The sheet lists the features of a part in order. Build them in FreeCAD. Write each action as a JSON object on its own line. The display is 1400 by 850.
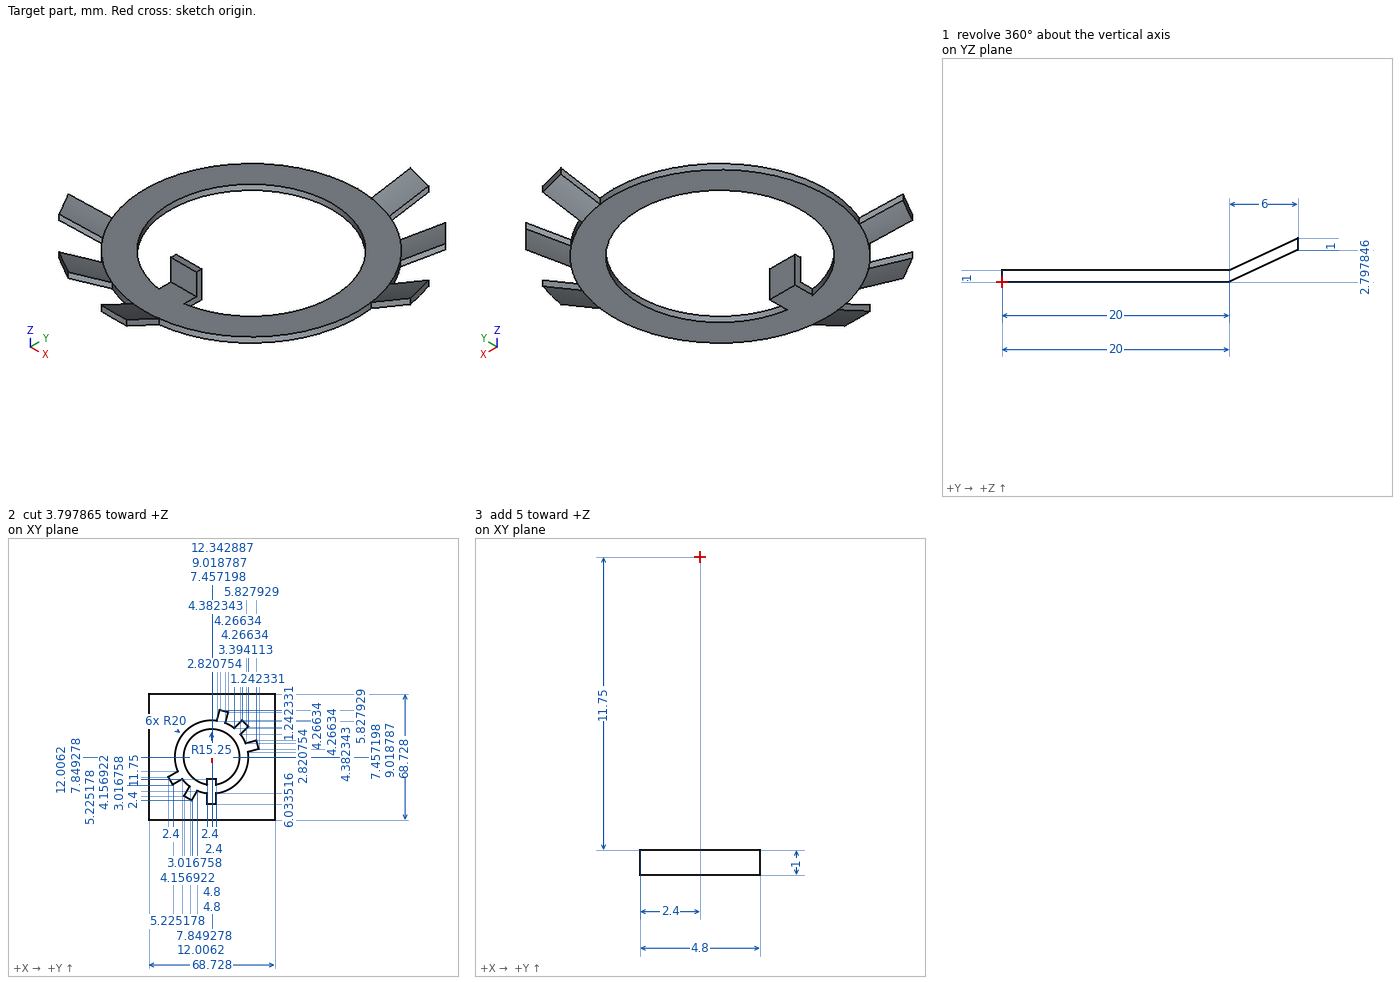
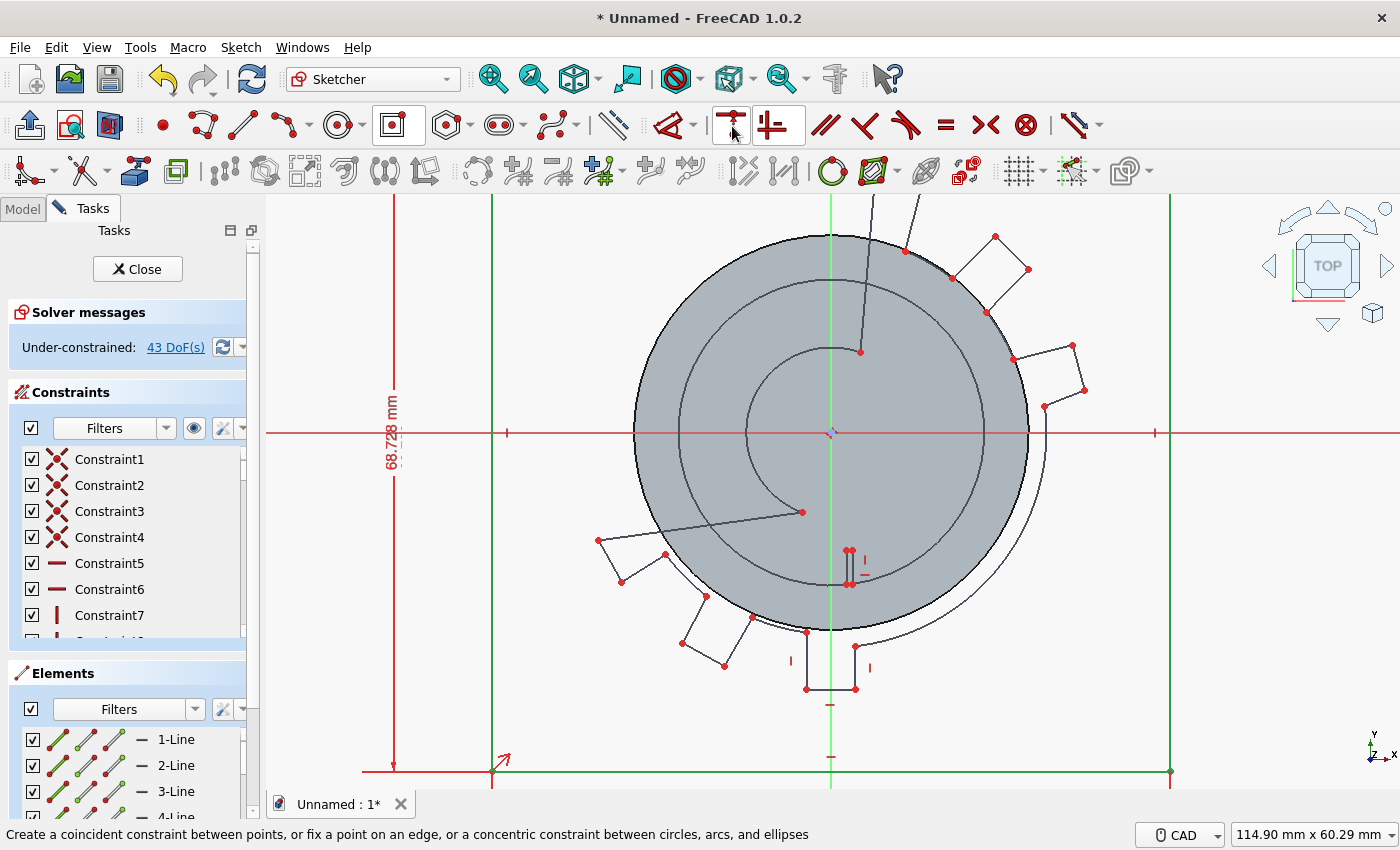
{"action": "left_click", "coordinate": [677, 568]}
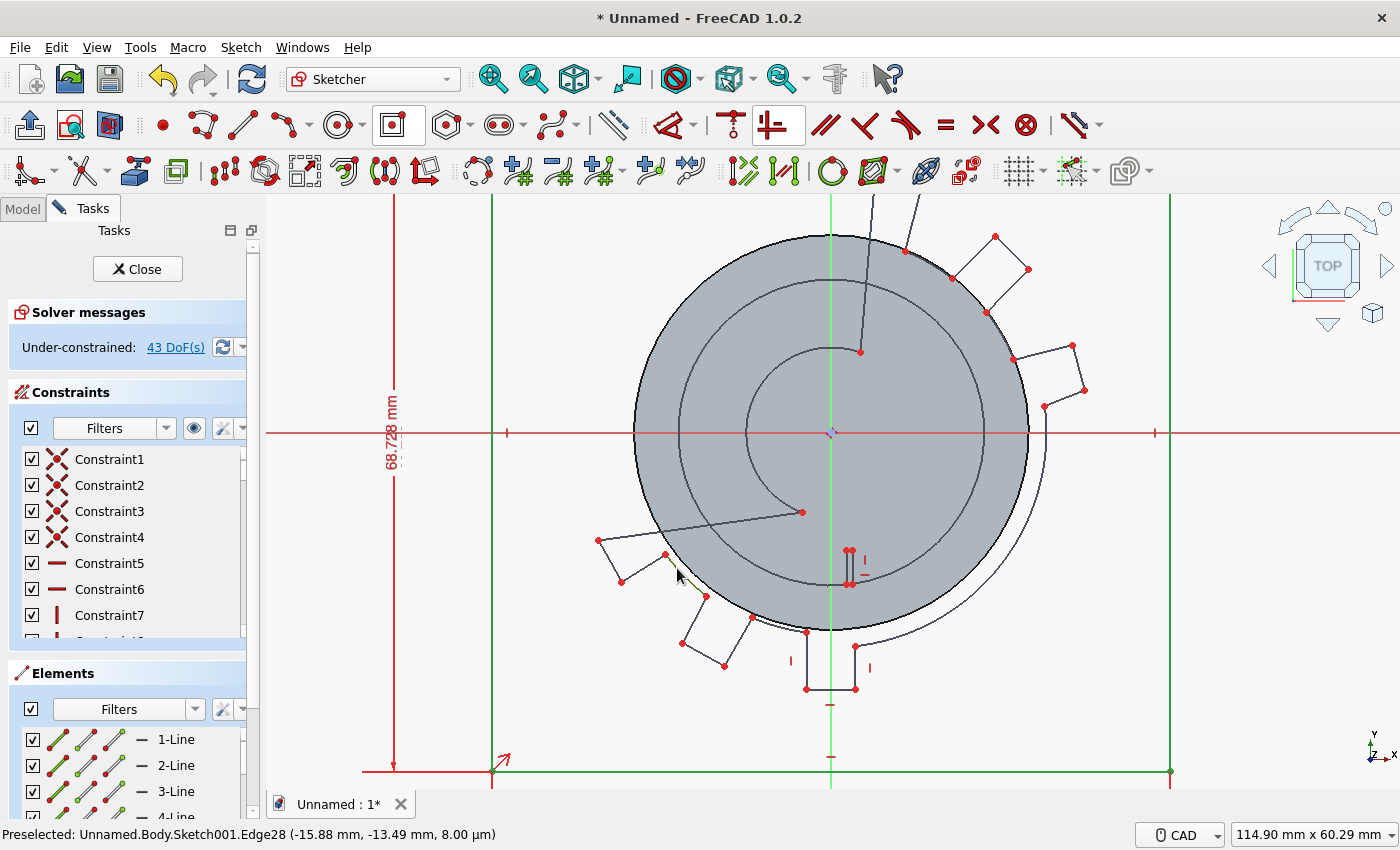
{"action": "left_click", "coordinate": [784, 362]}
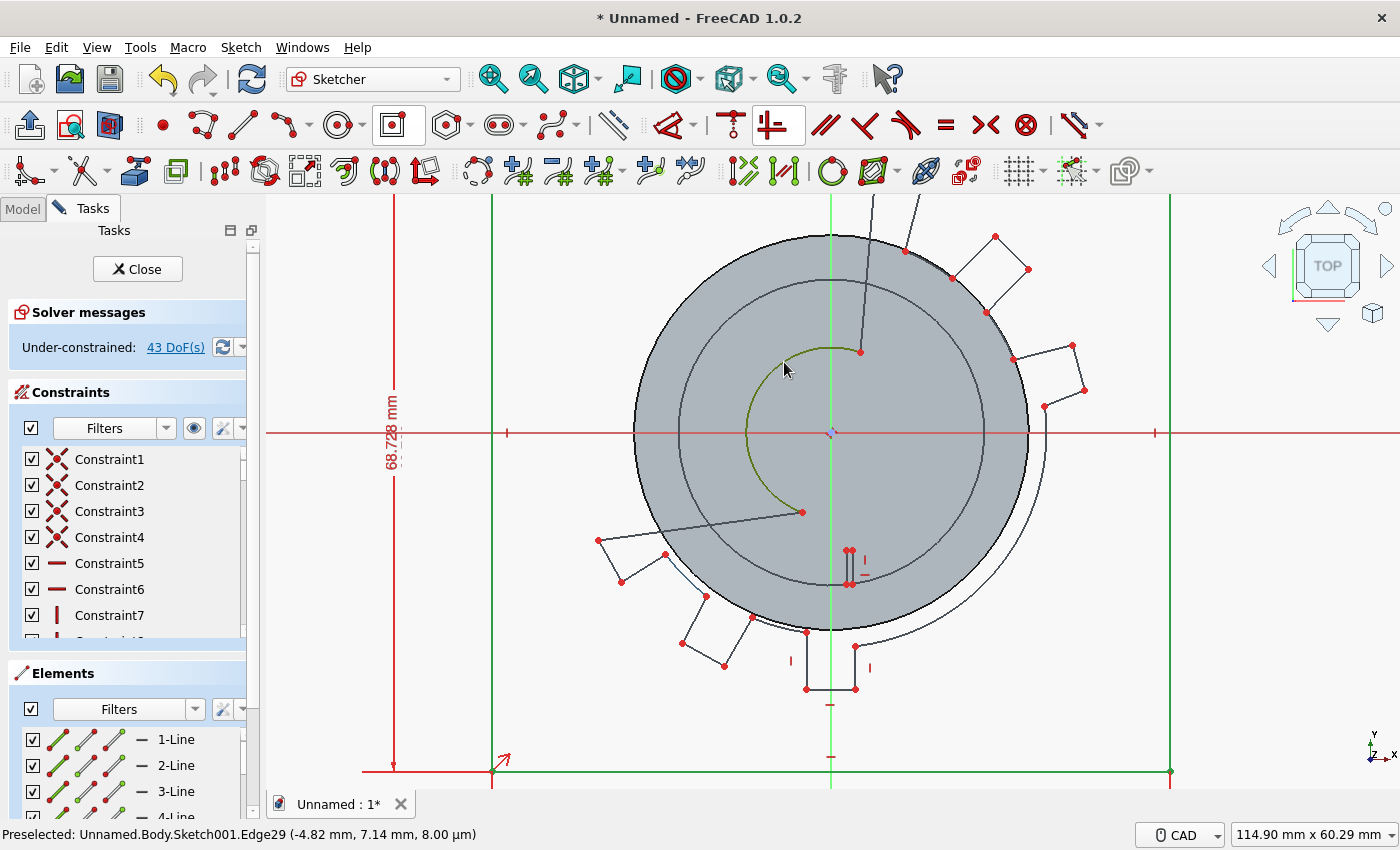
{"action": "left_click", "coordinate": [939, 269]}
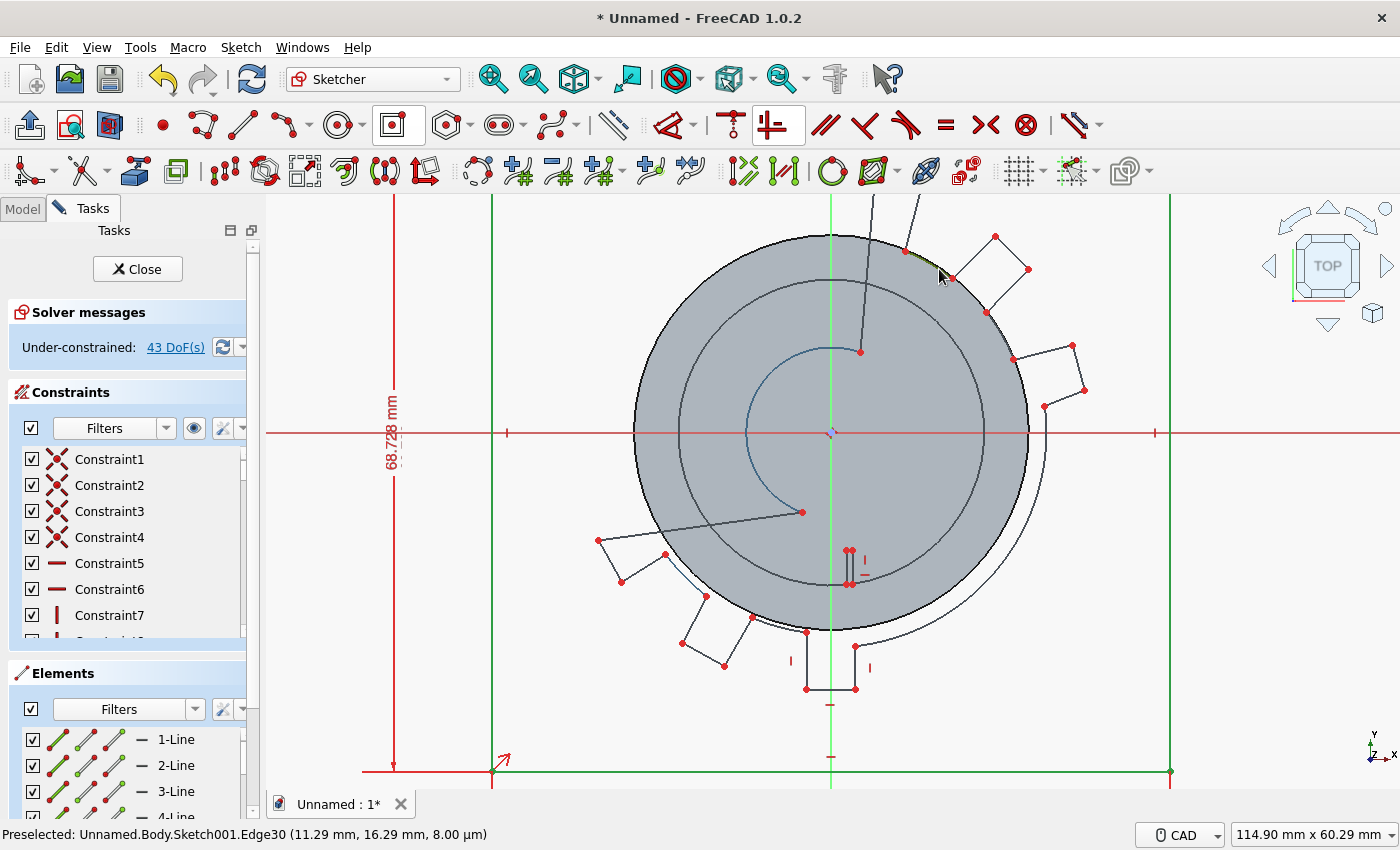
{"action": "left_click", "coordinate": [1007, 345]}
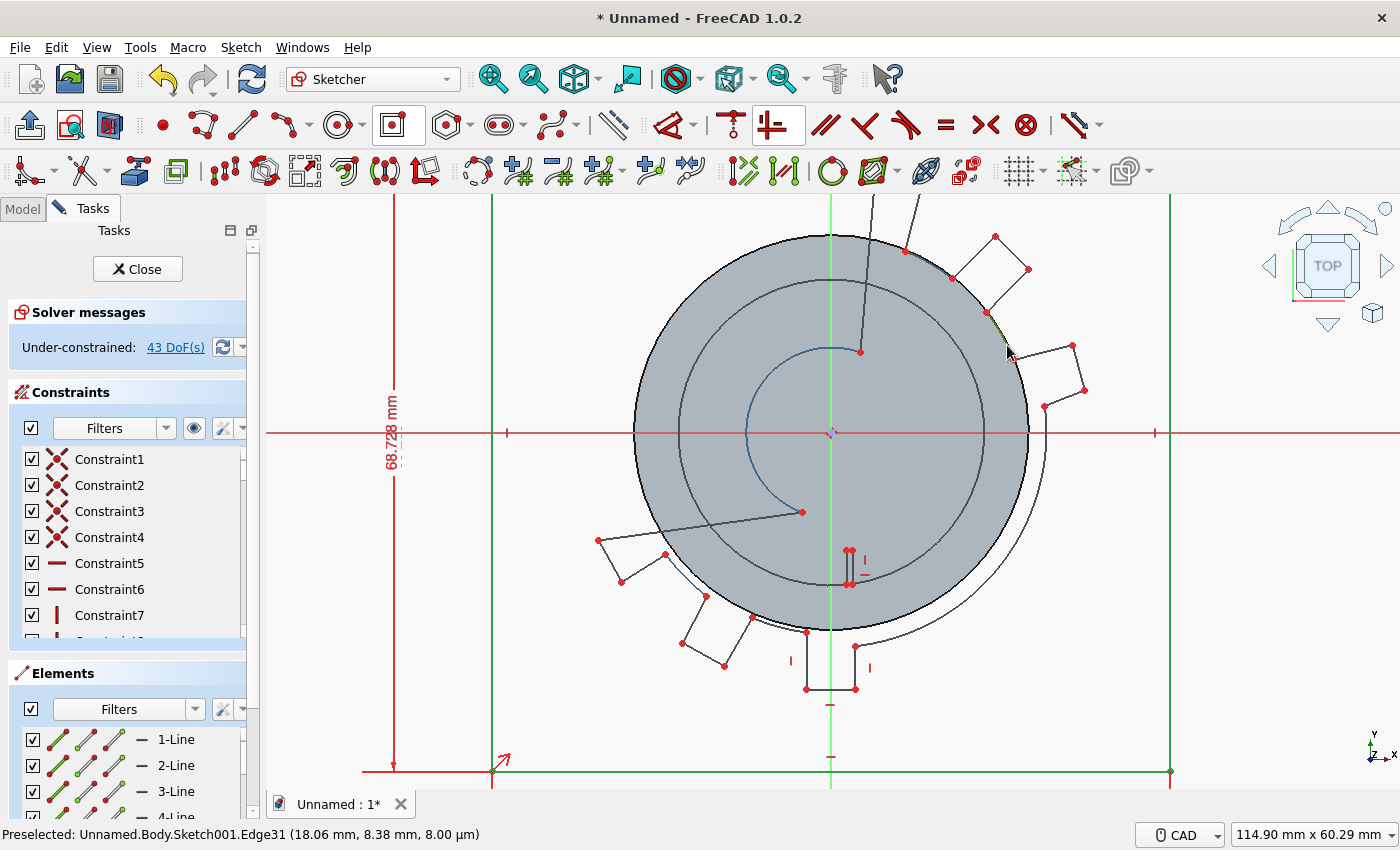
{"action": "left_click", "coordinate": [950, 612]}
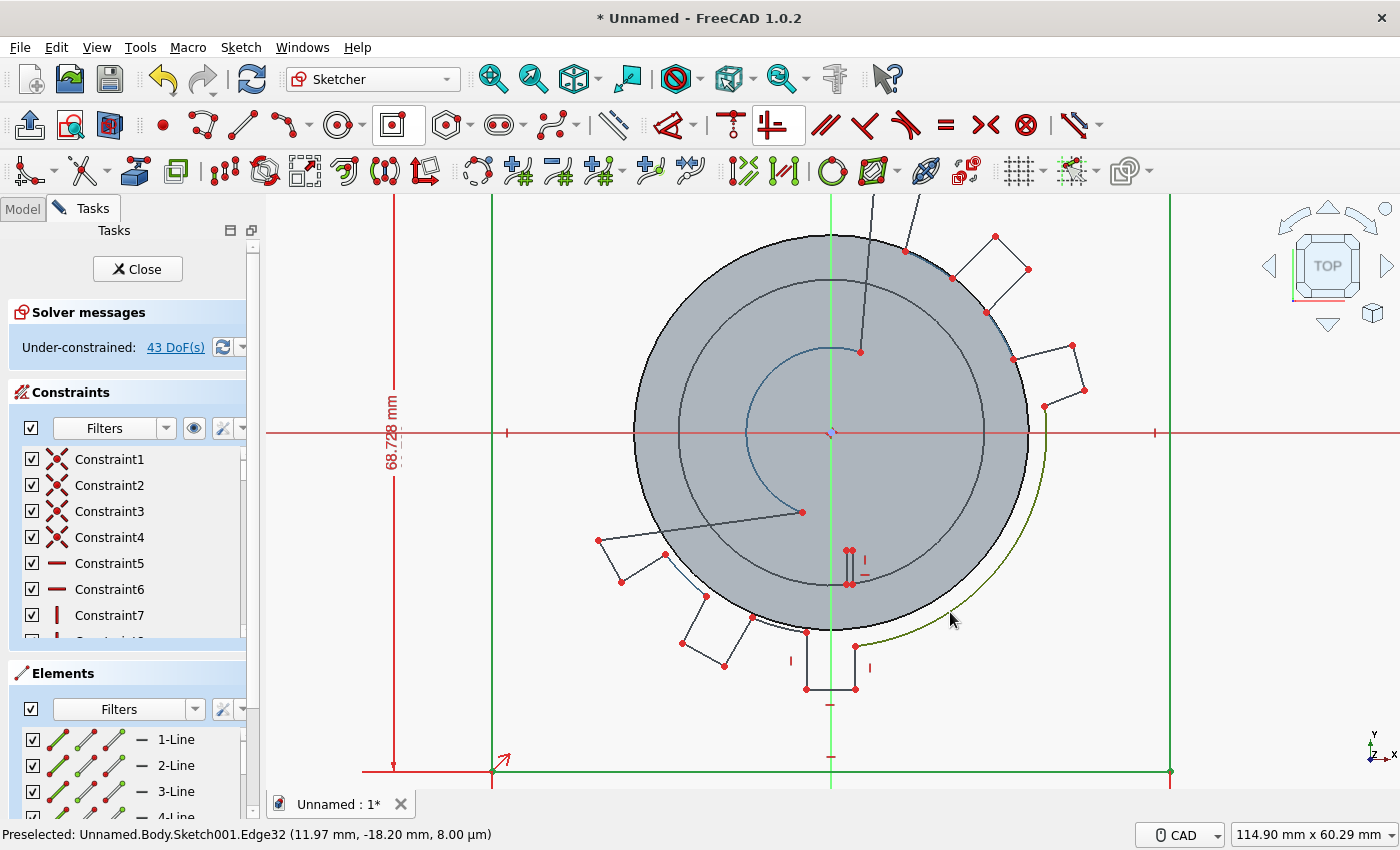
{"action": "left_click", "coordinate": [768, 624]}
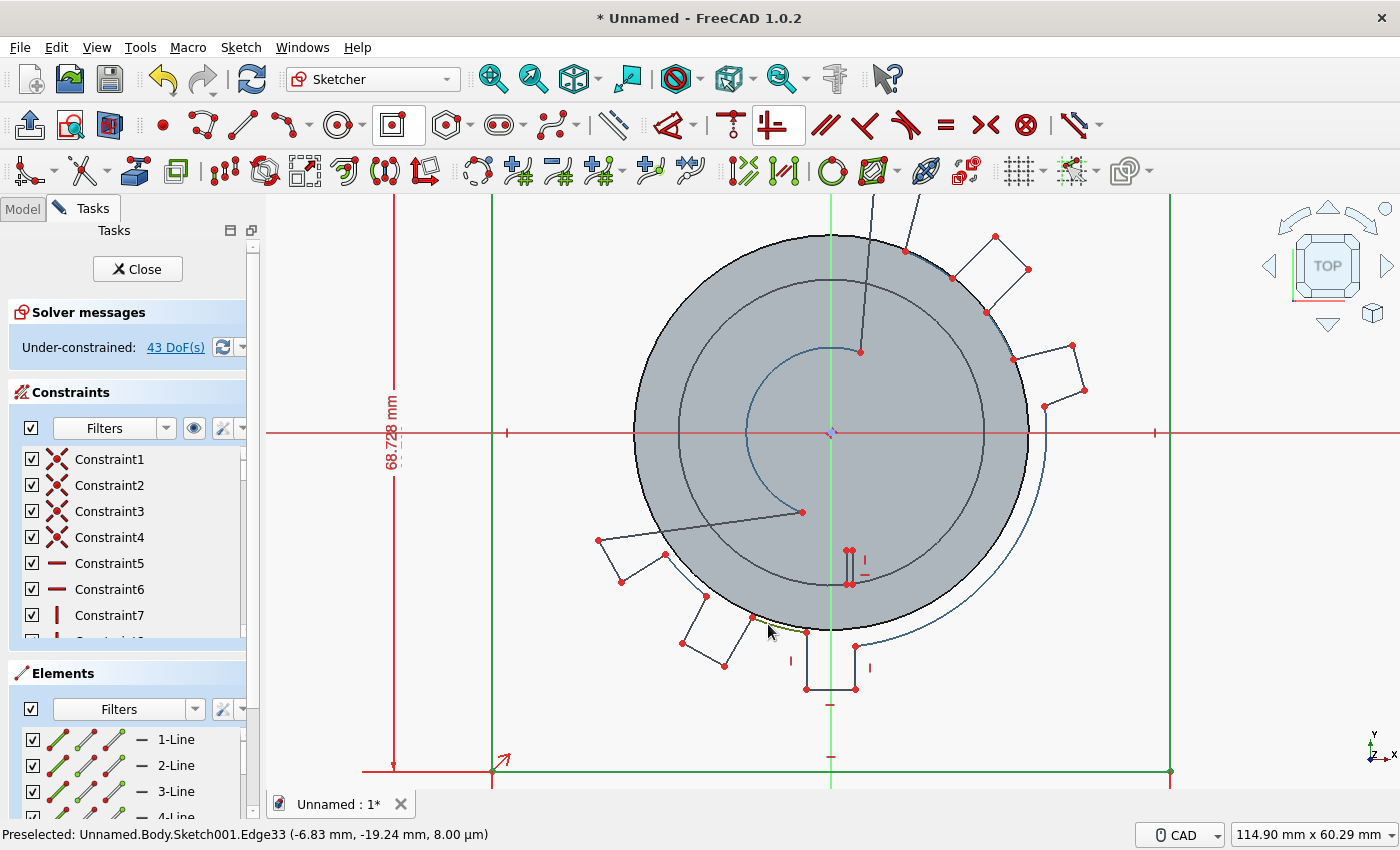
{"action": "left_click", "coordinate": [946, 126]}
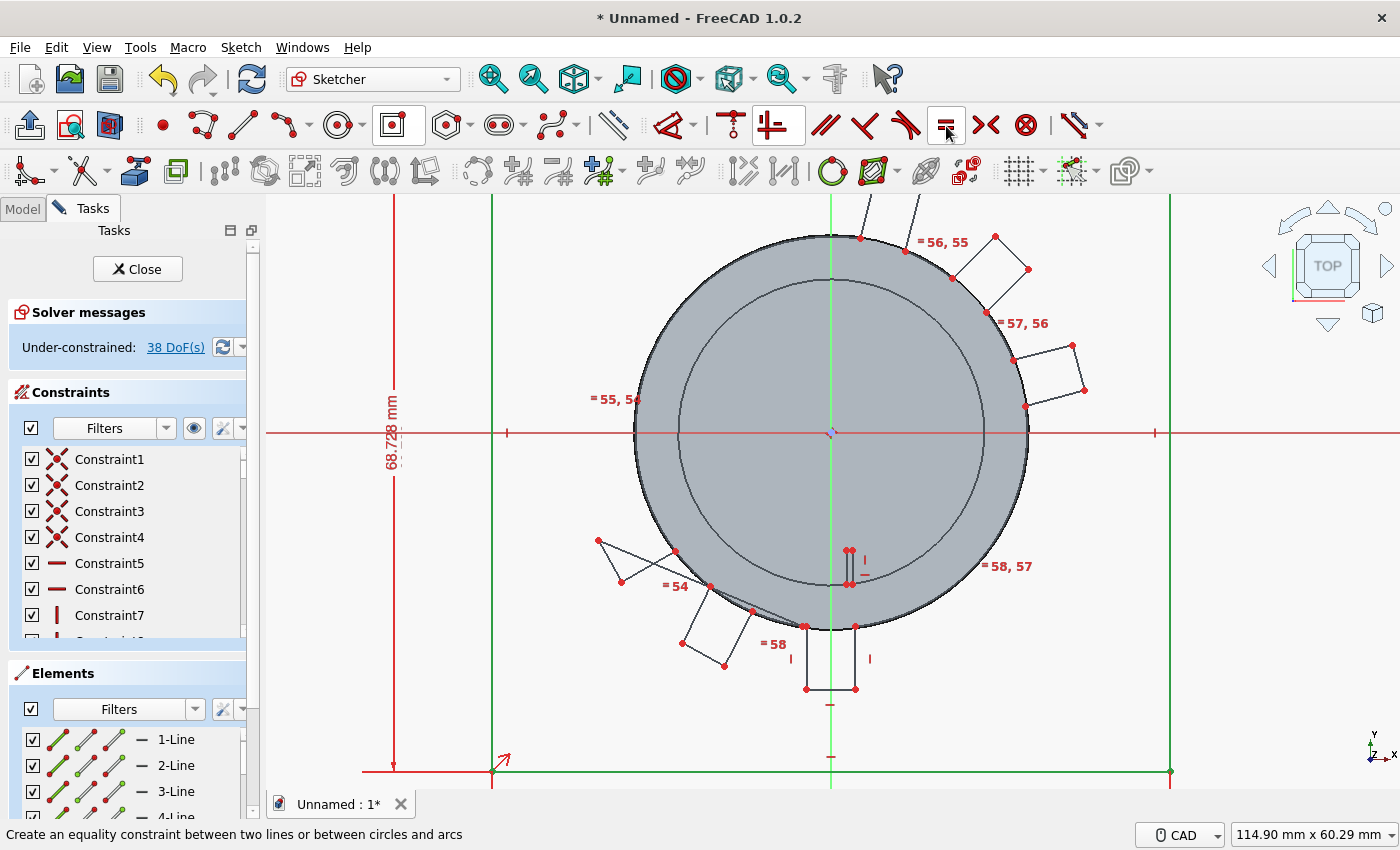
{"action": "left_click", "coordinate": [668, 126]}